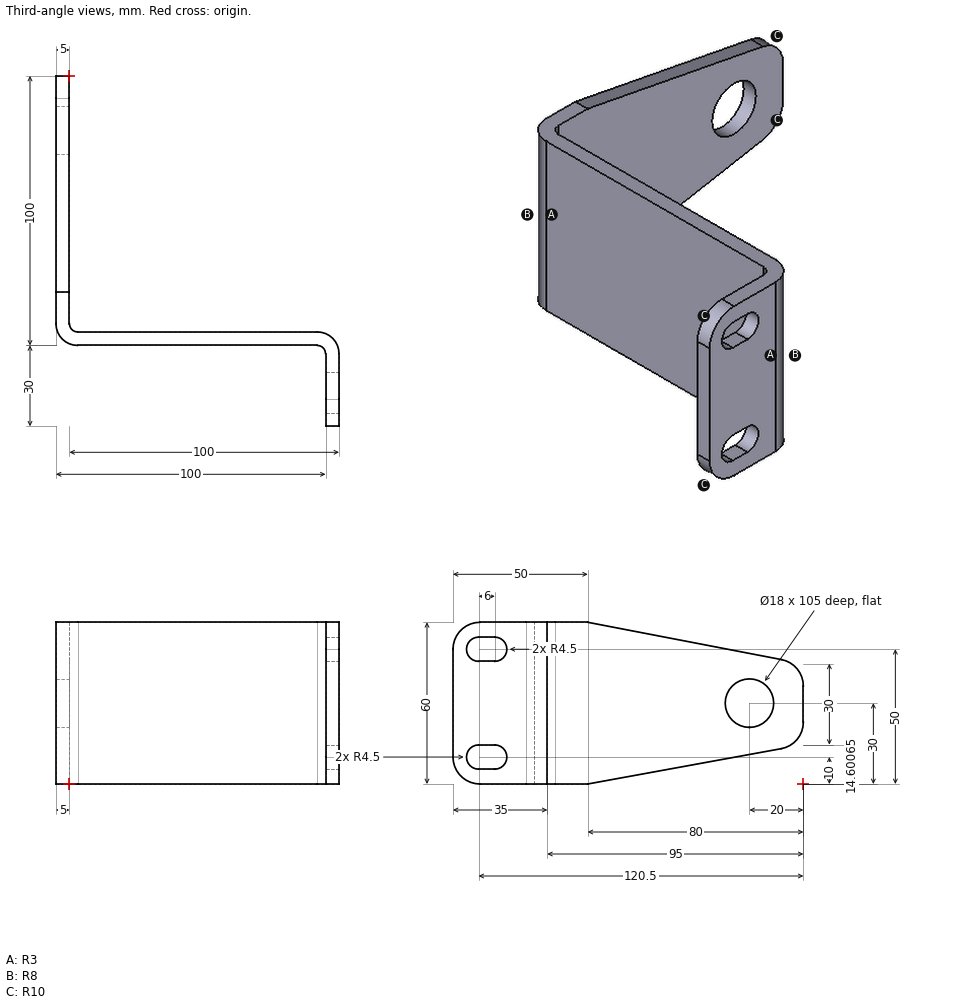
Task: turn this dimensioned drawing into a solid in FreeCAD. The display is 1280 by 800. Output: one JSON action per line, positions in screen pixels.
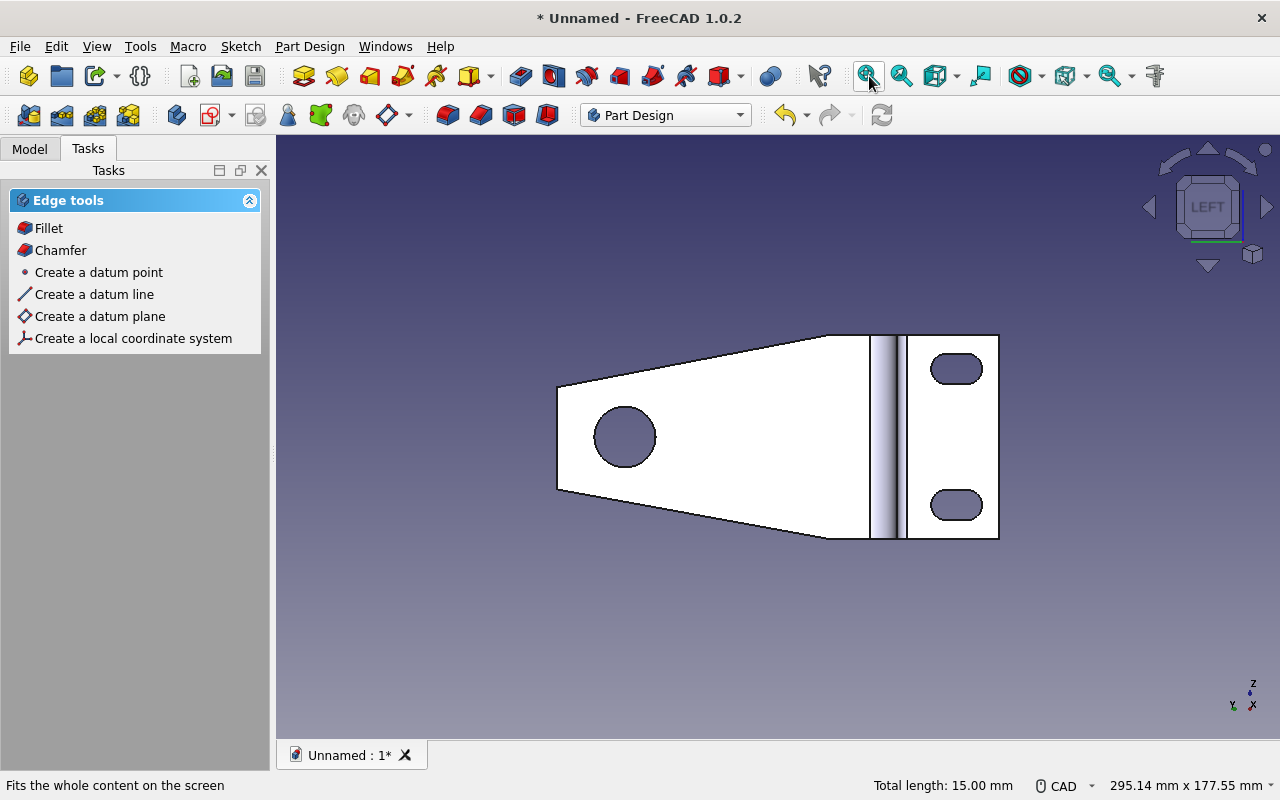
{"action": "key", "text": "v 3"}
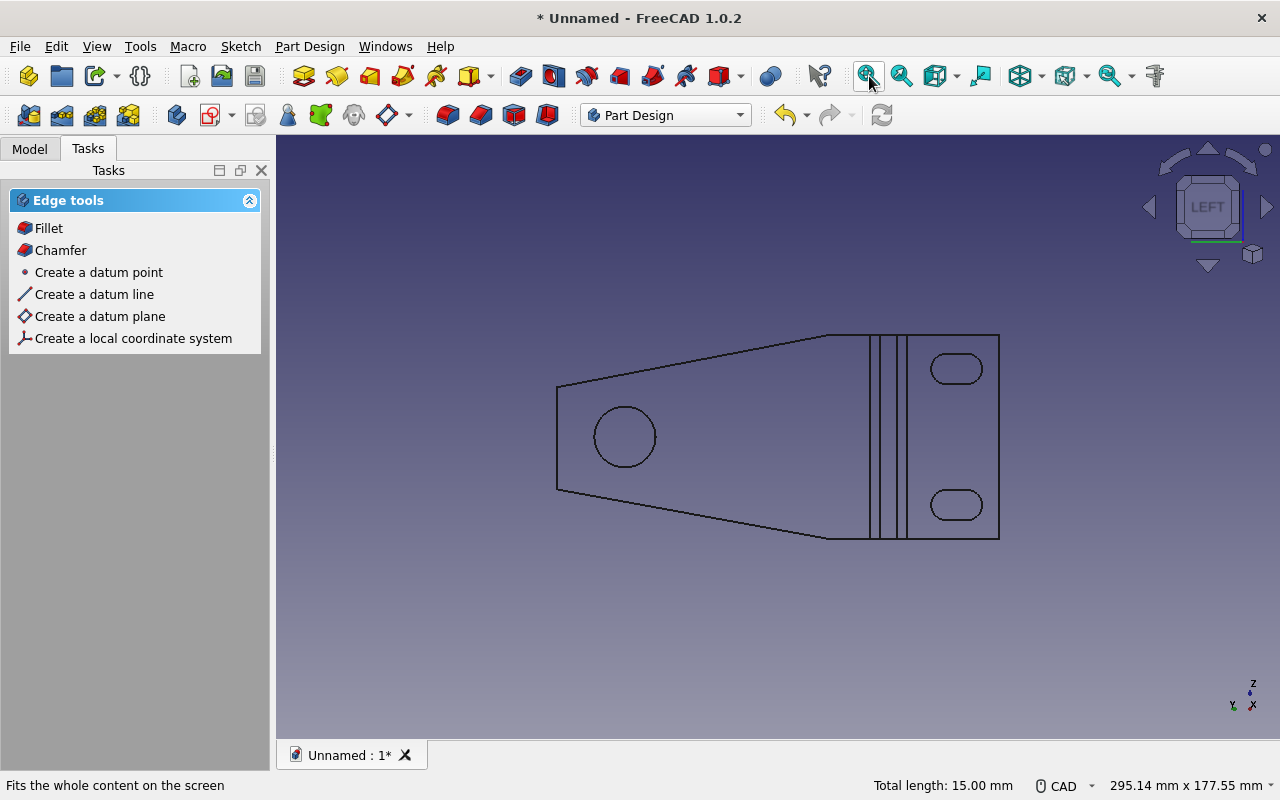
{"action": "key", "text": "0"}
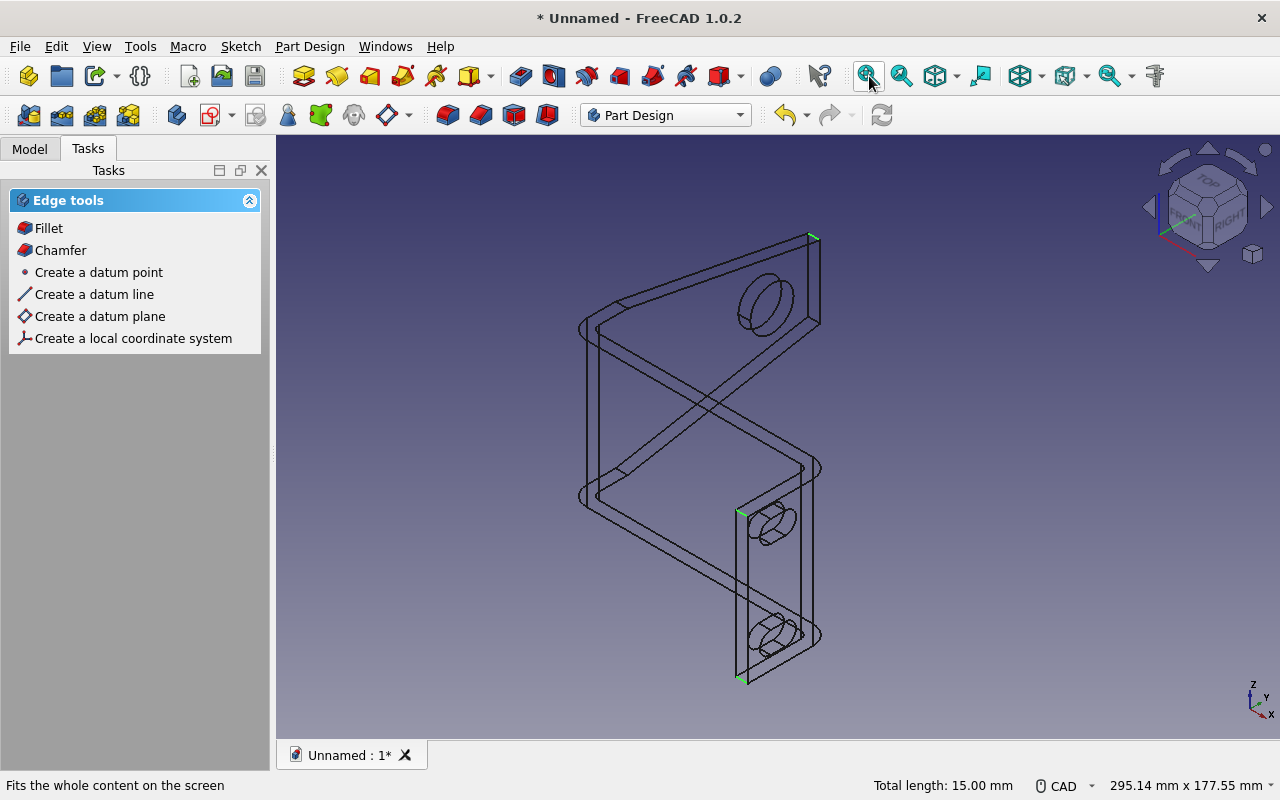
{"action": "left_click", "coordinate": [814, 319], "text": "ctrl"}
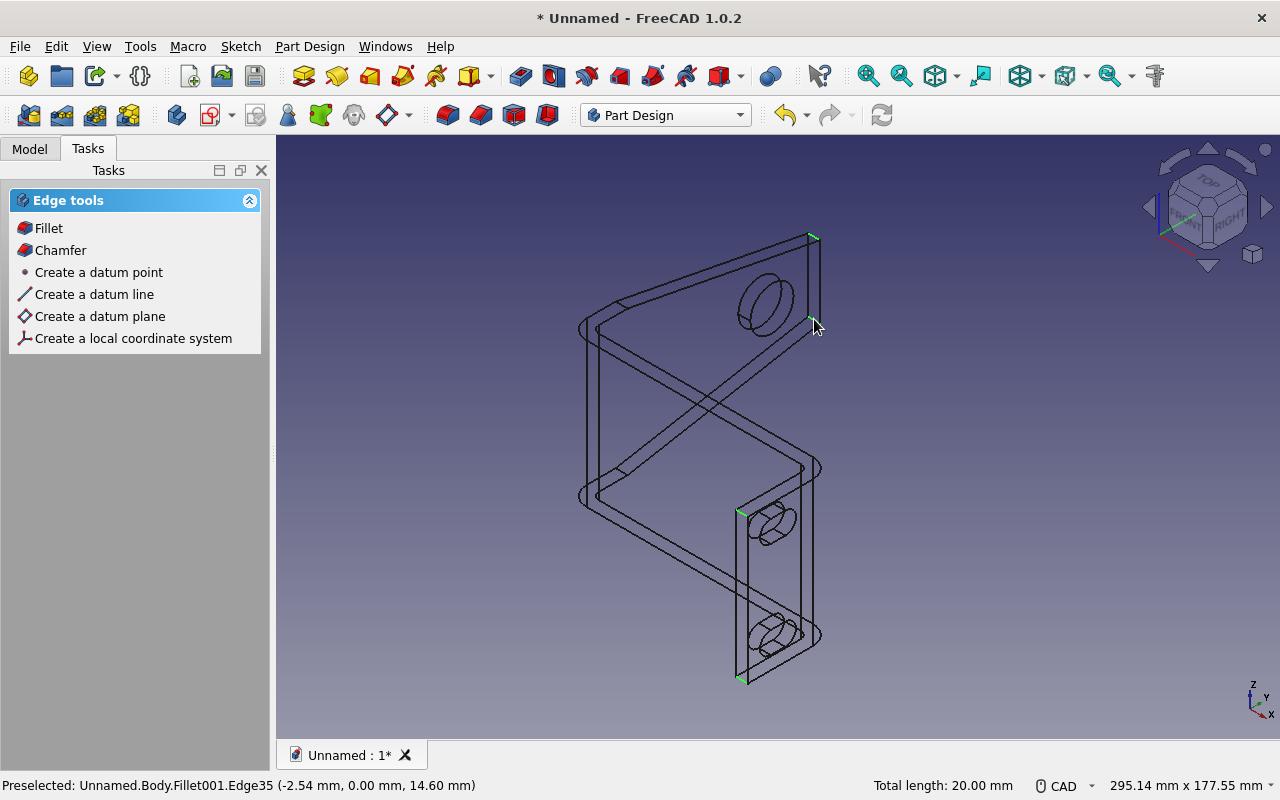
{"action": "key", "text": "v 1"}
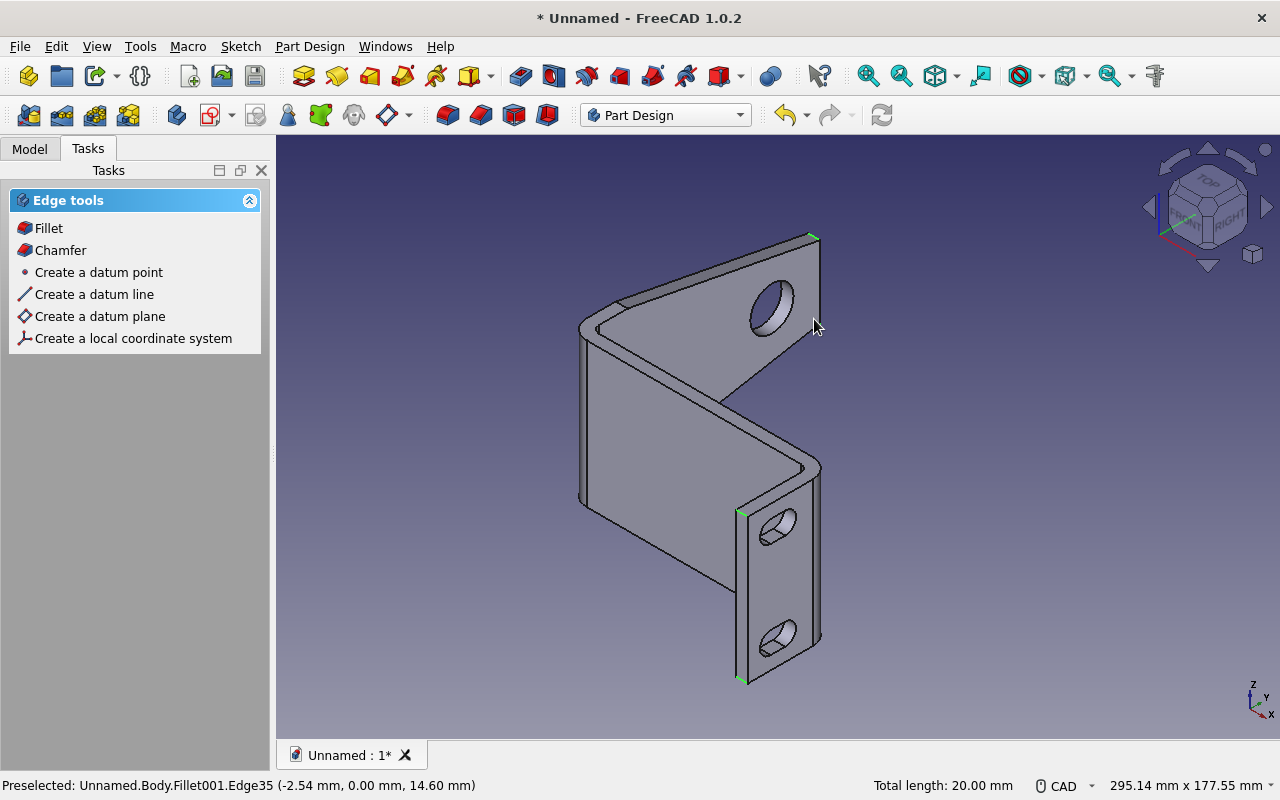
{"action": "left_click", "coordinate": [448, 116]}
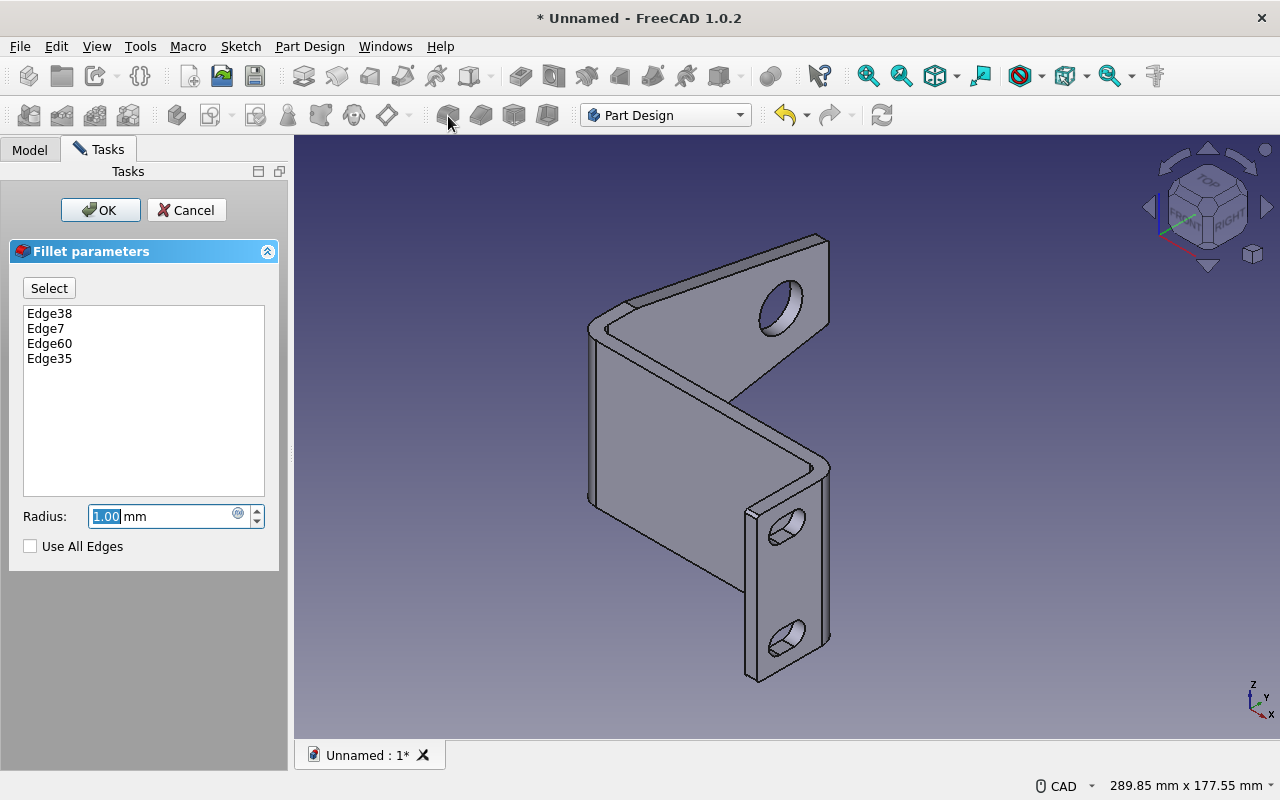
{"action": "type", "text": "10"}
{"action": "key", "text": "Tab"}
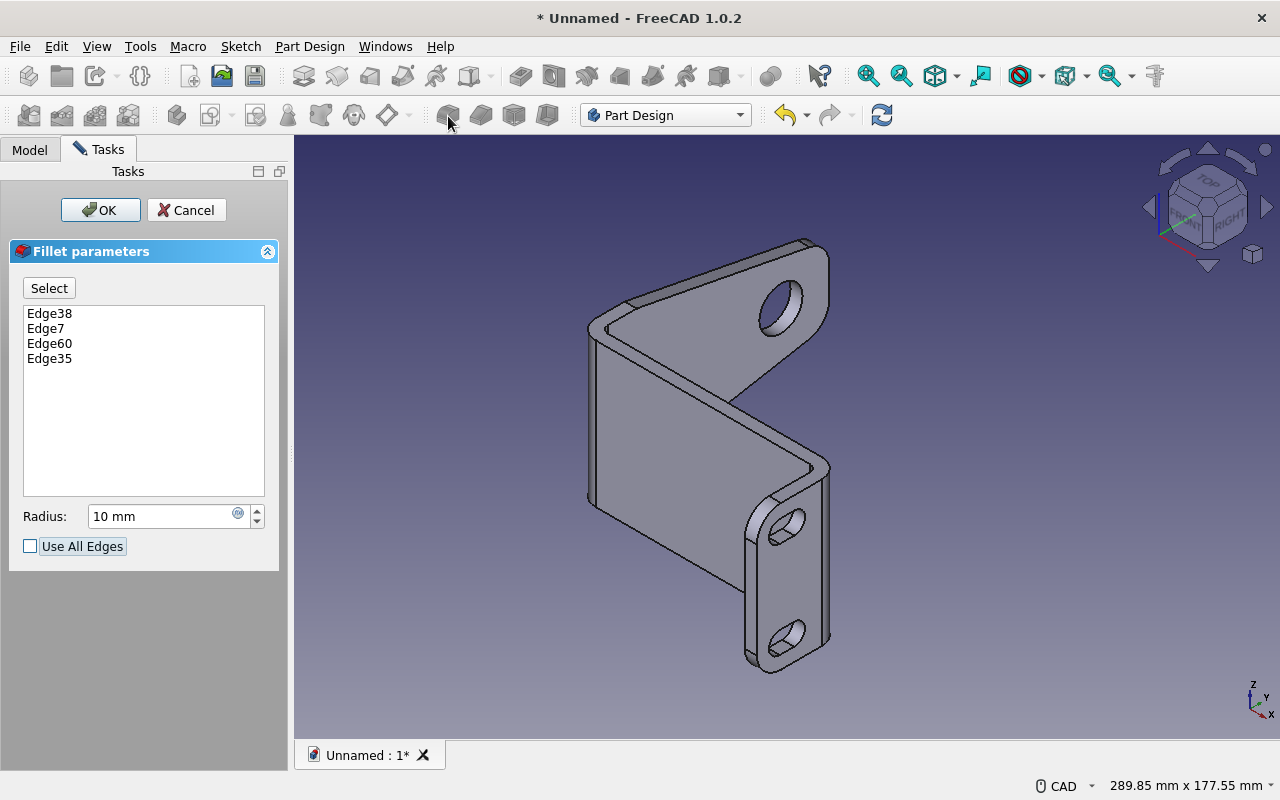
{"action": "left_click", "coordinate": [101, 210]}